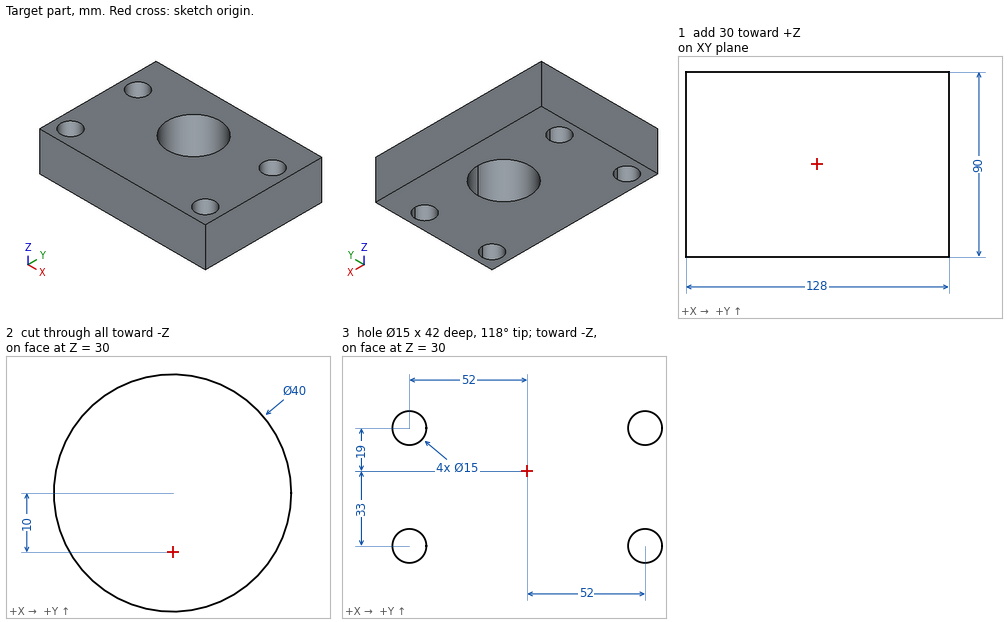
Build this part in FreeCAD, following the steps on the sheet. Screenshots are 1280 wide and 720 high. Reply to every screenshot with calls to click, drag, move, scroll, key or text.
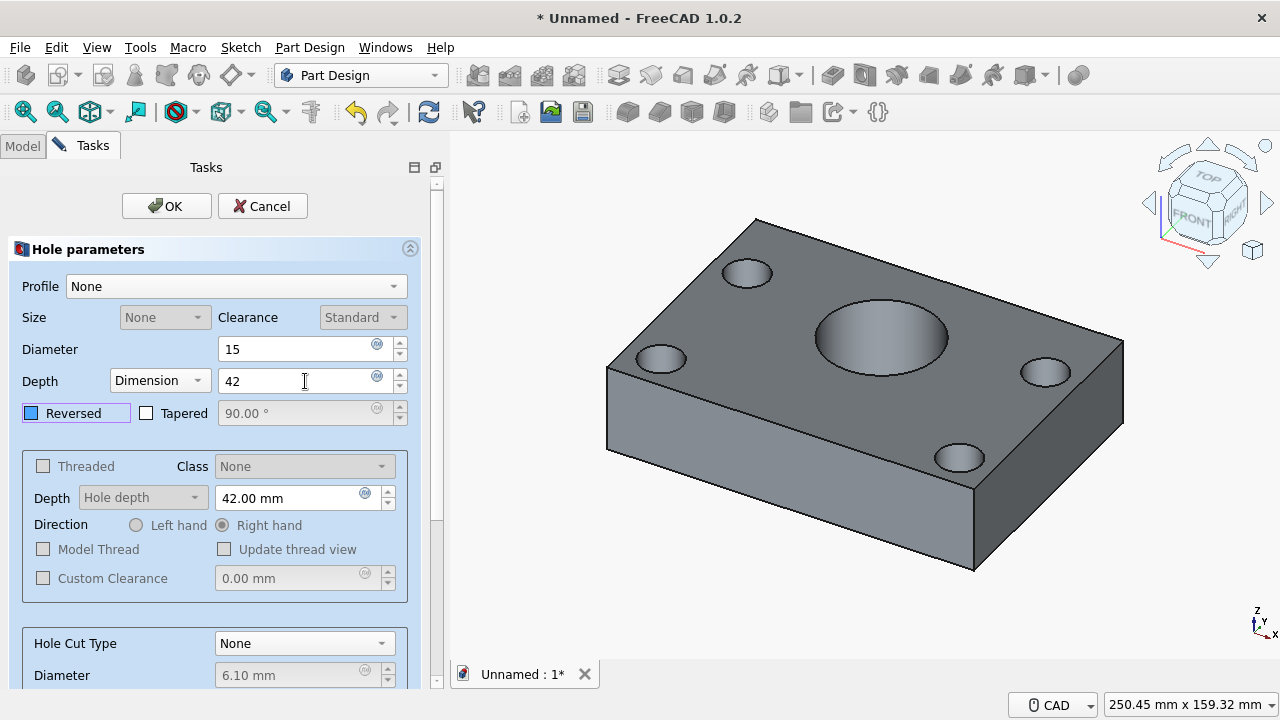
click(167, 206)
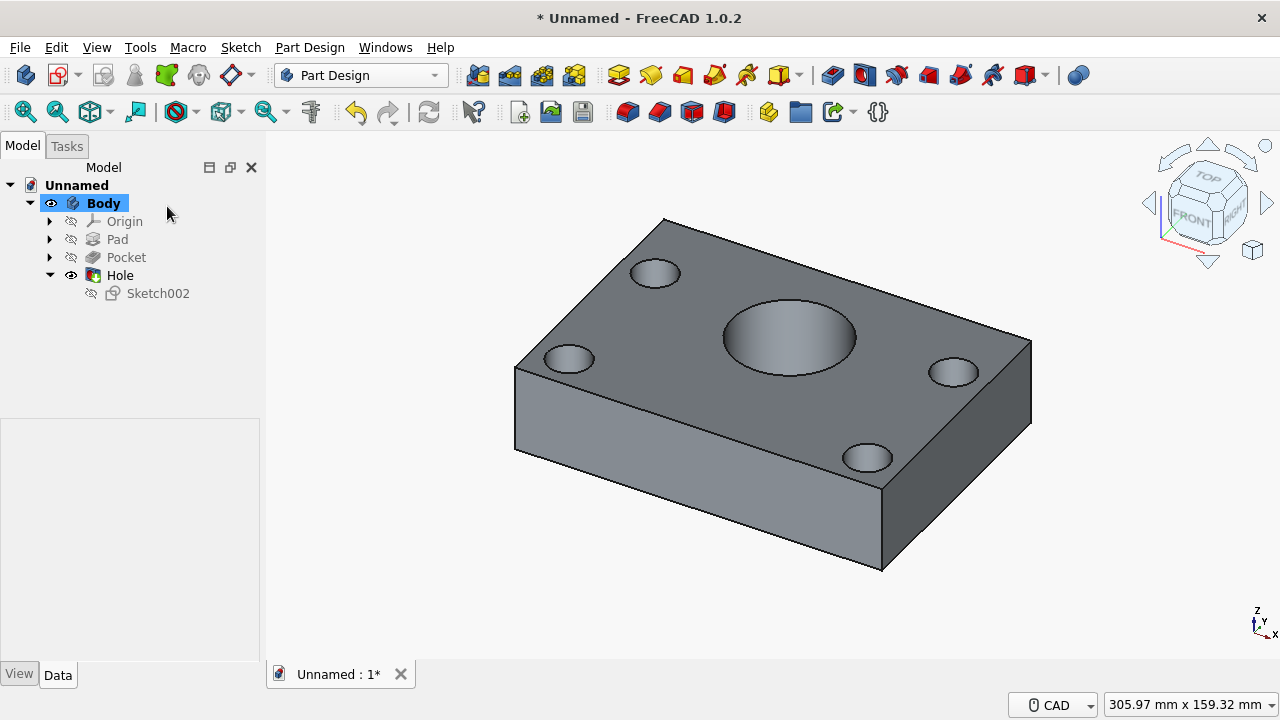
key(0)